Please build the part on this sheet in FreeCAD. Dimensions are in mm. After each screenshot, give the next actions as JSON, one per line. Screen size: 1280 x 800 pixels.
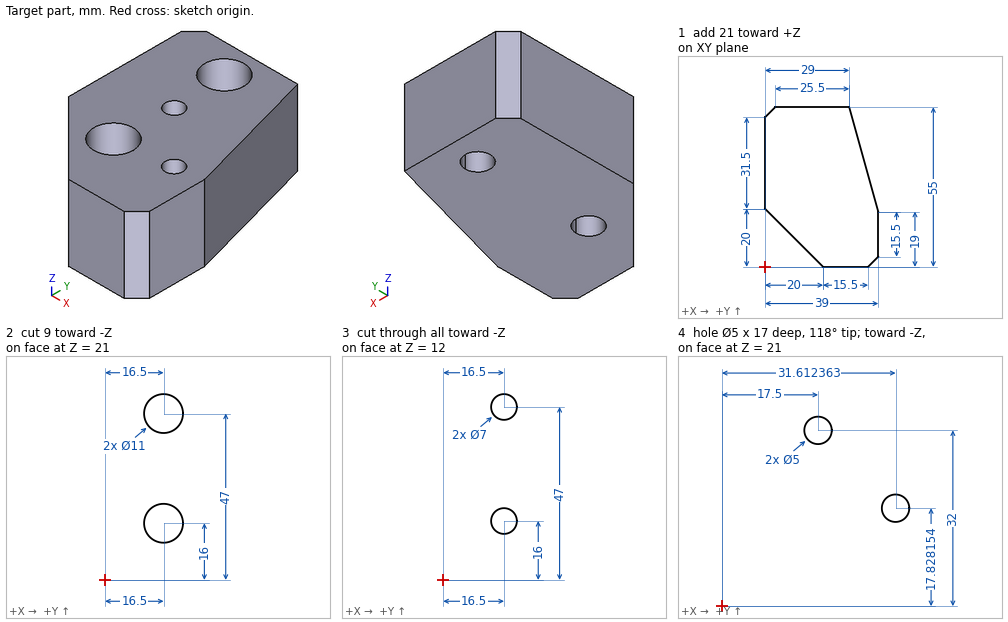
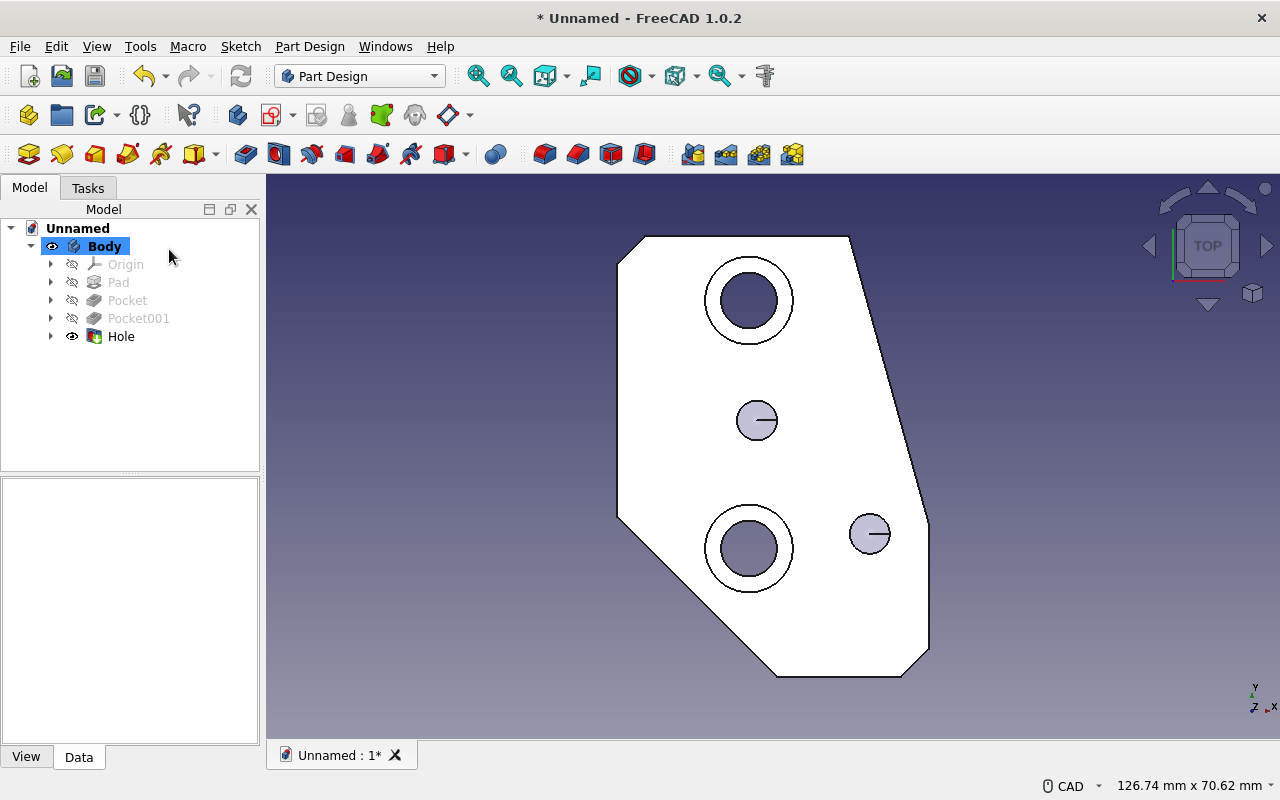
{"action": "key", "text": "0"}